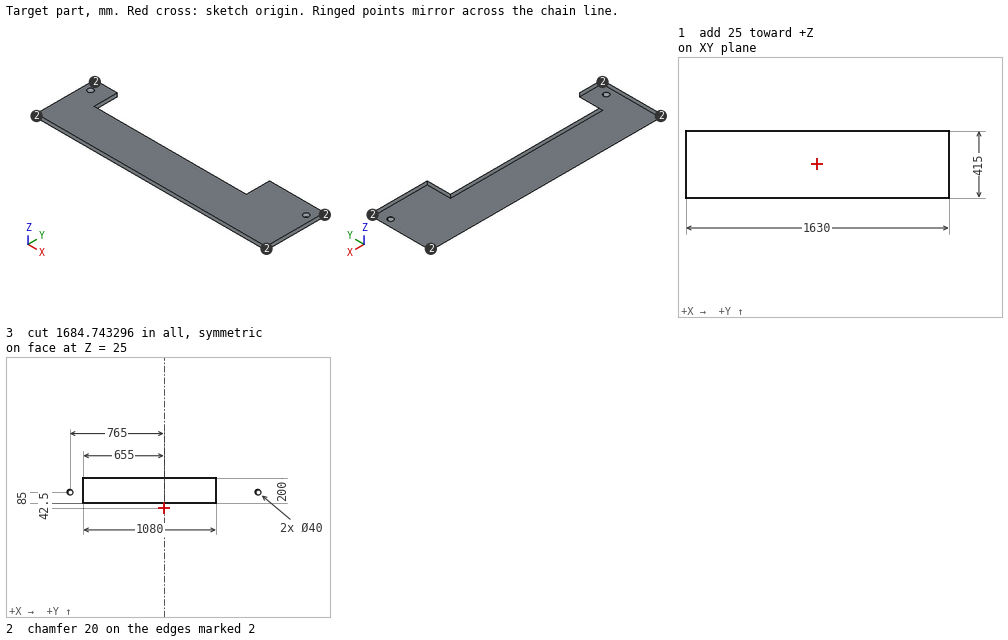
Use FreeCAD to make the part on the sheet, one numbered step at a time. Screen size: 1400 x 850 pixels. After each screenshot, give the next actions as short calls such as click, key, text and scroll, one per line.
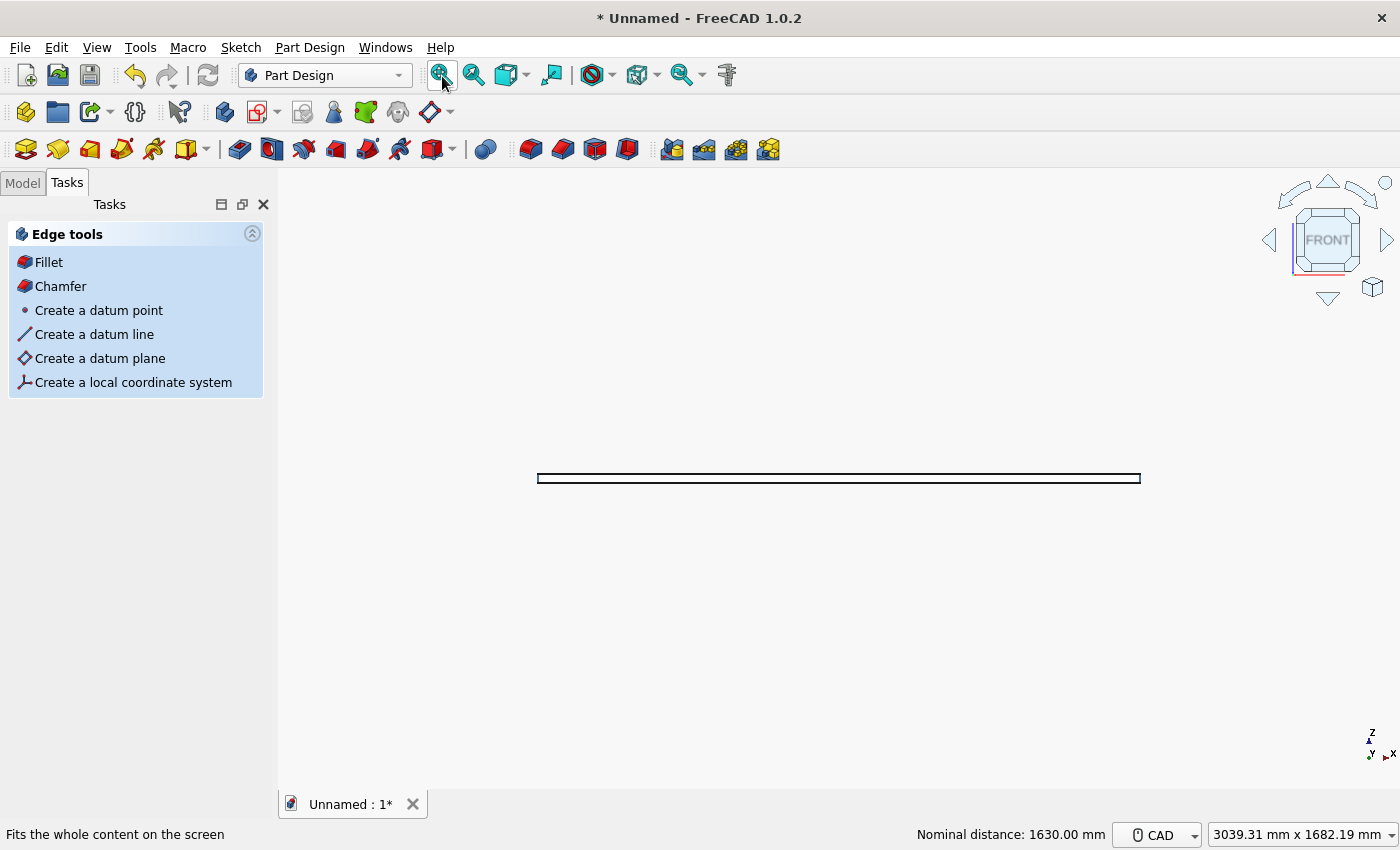
key(3)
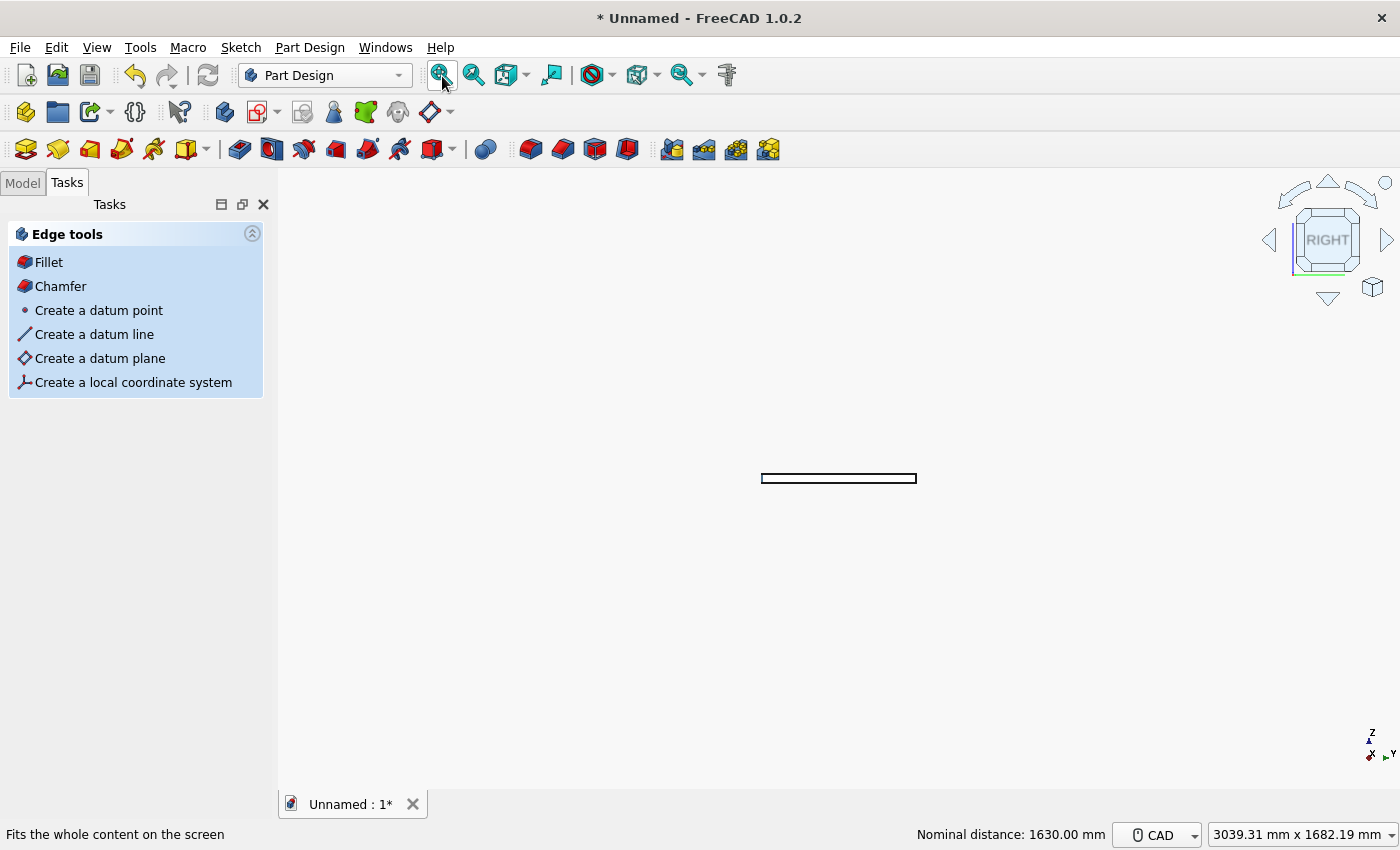
click(442, 76)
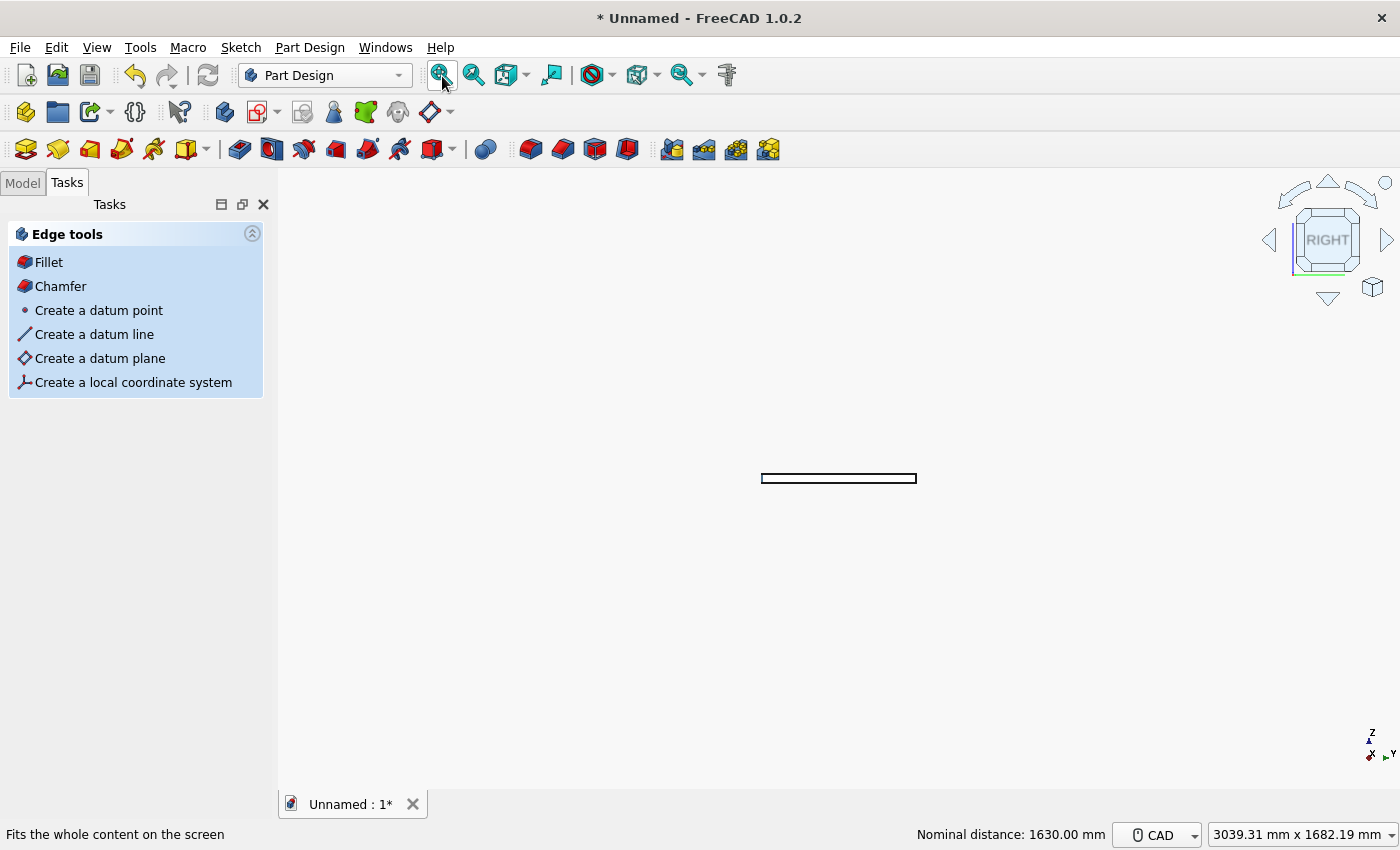
scroll(916, 477, up, 8)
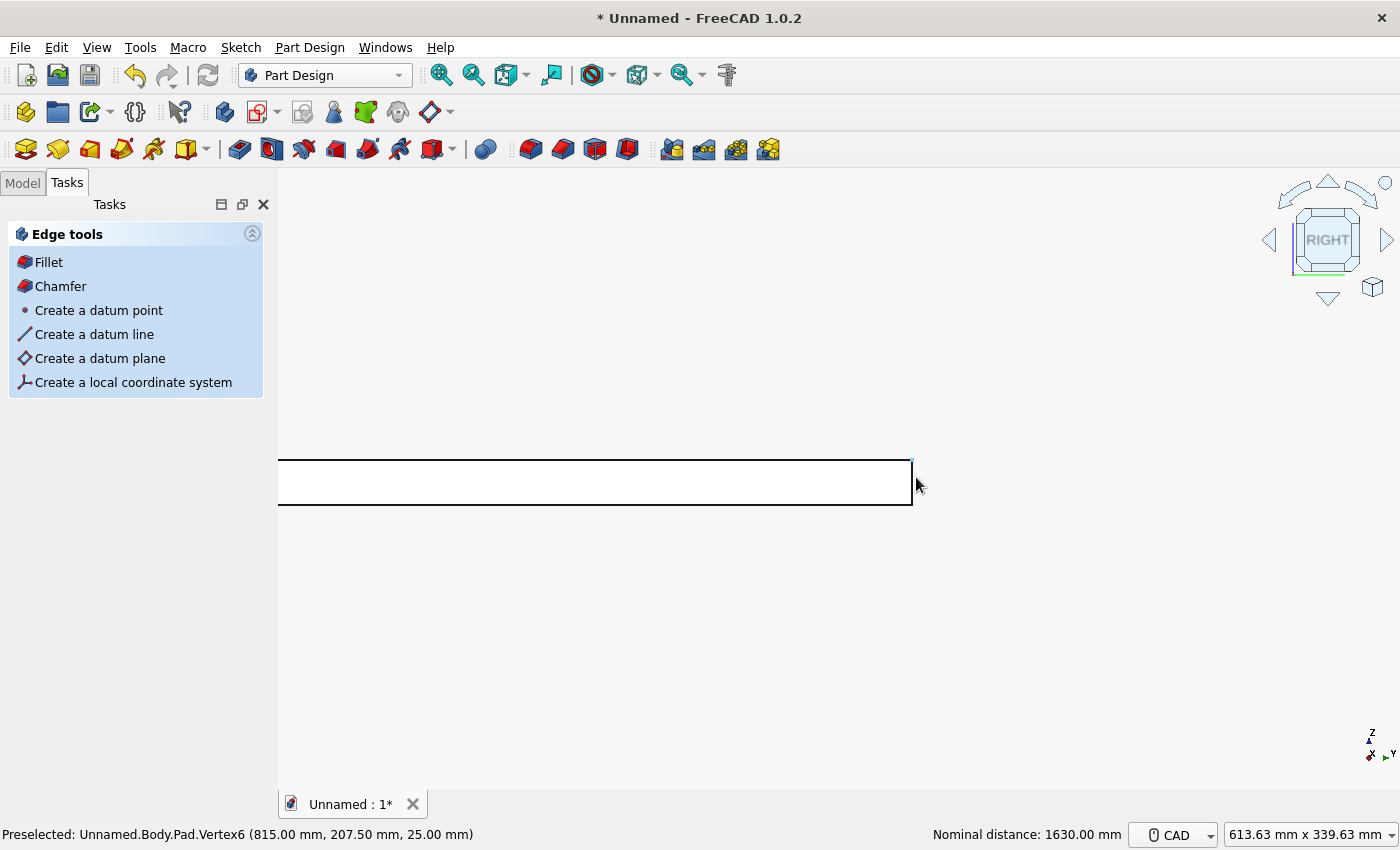
click(912, 481, ctrl)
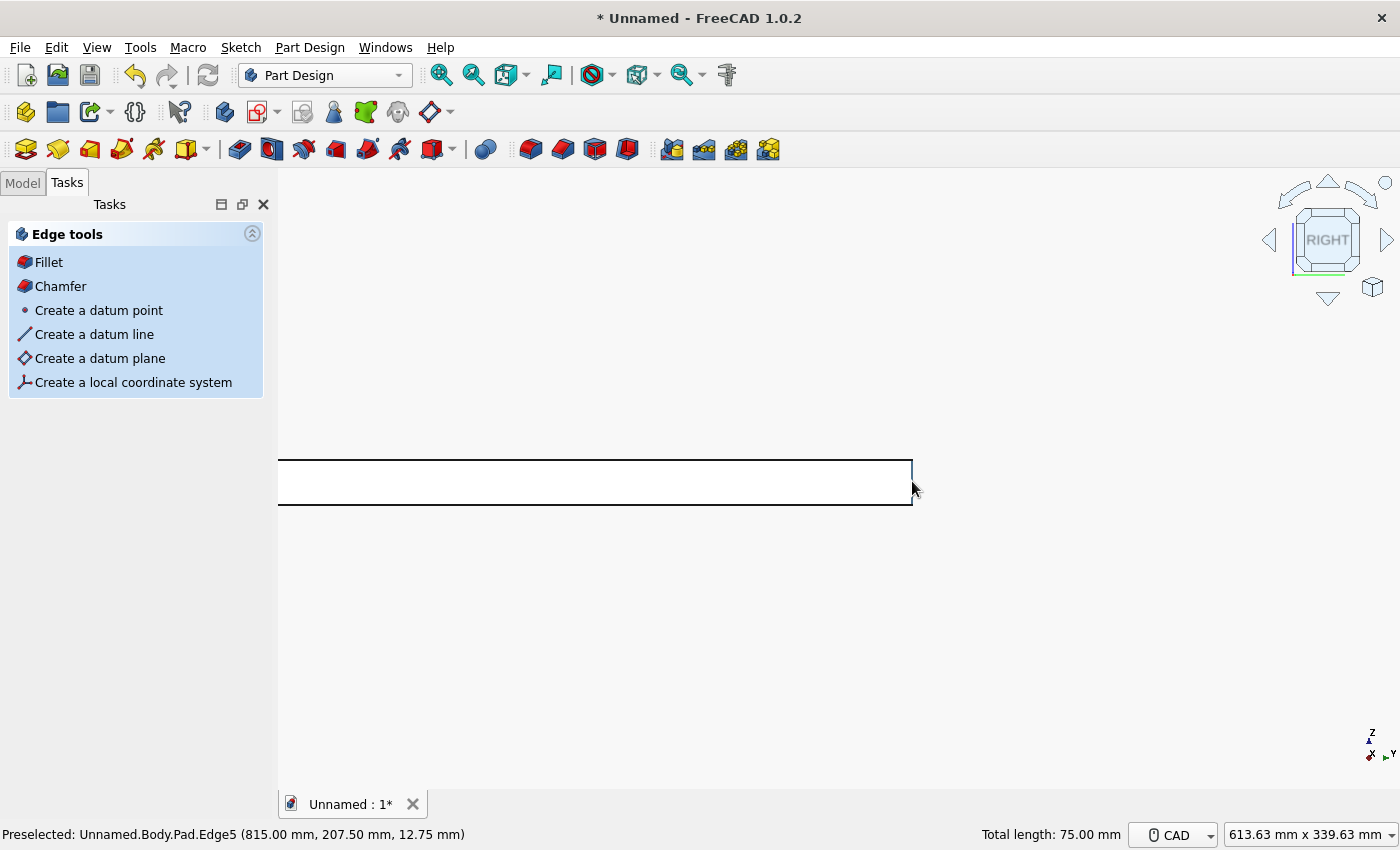
click(442, 76)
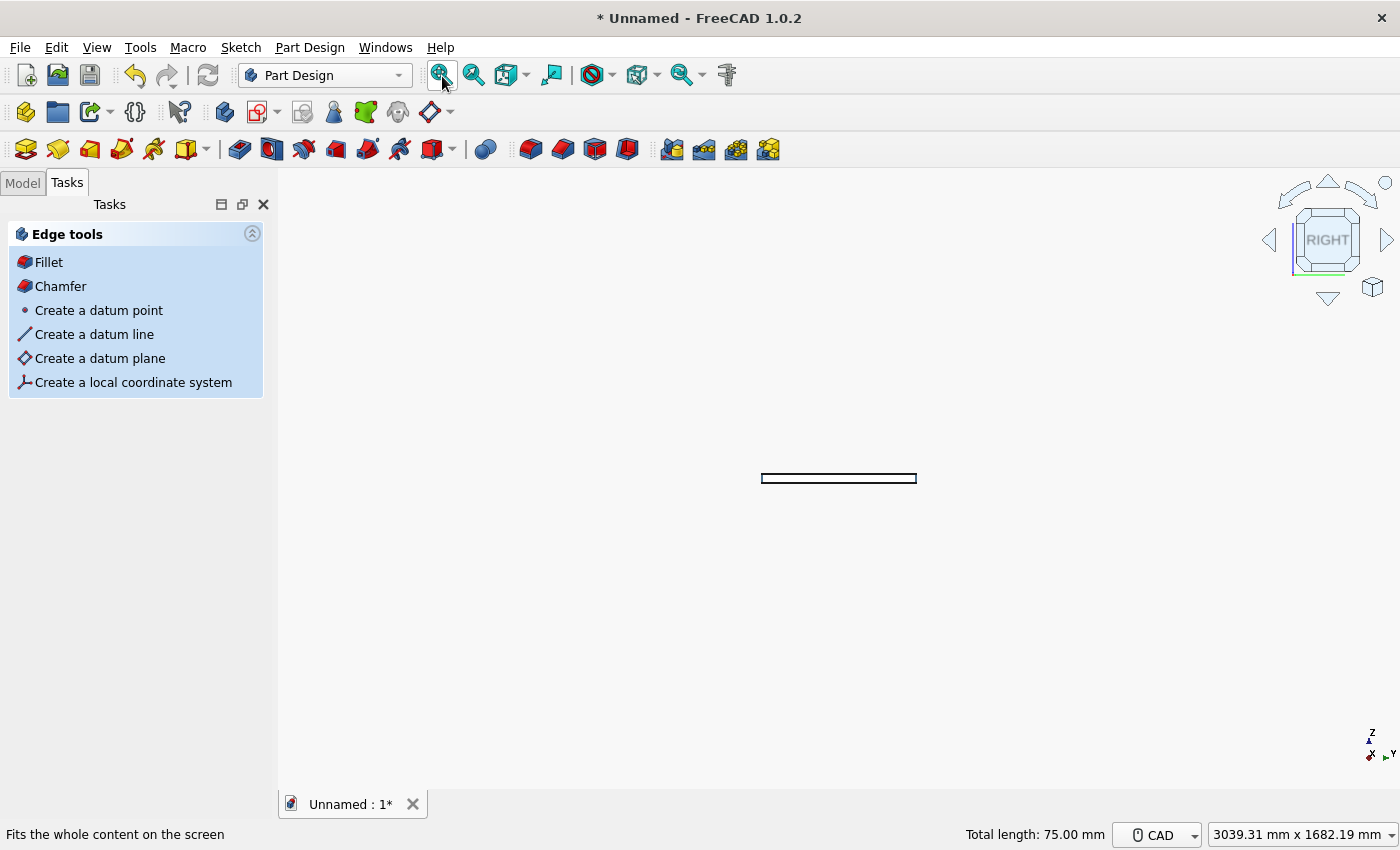
key(5)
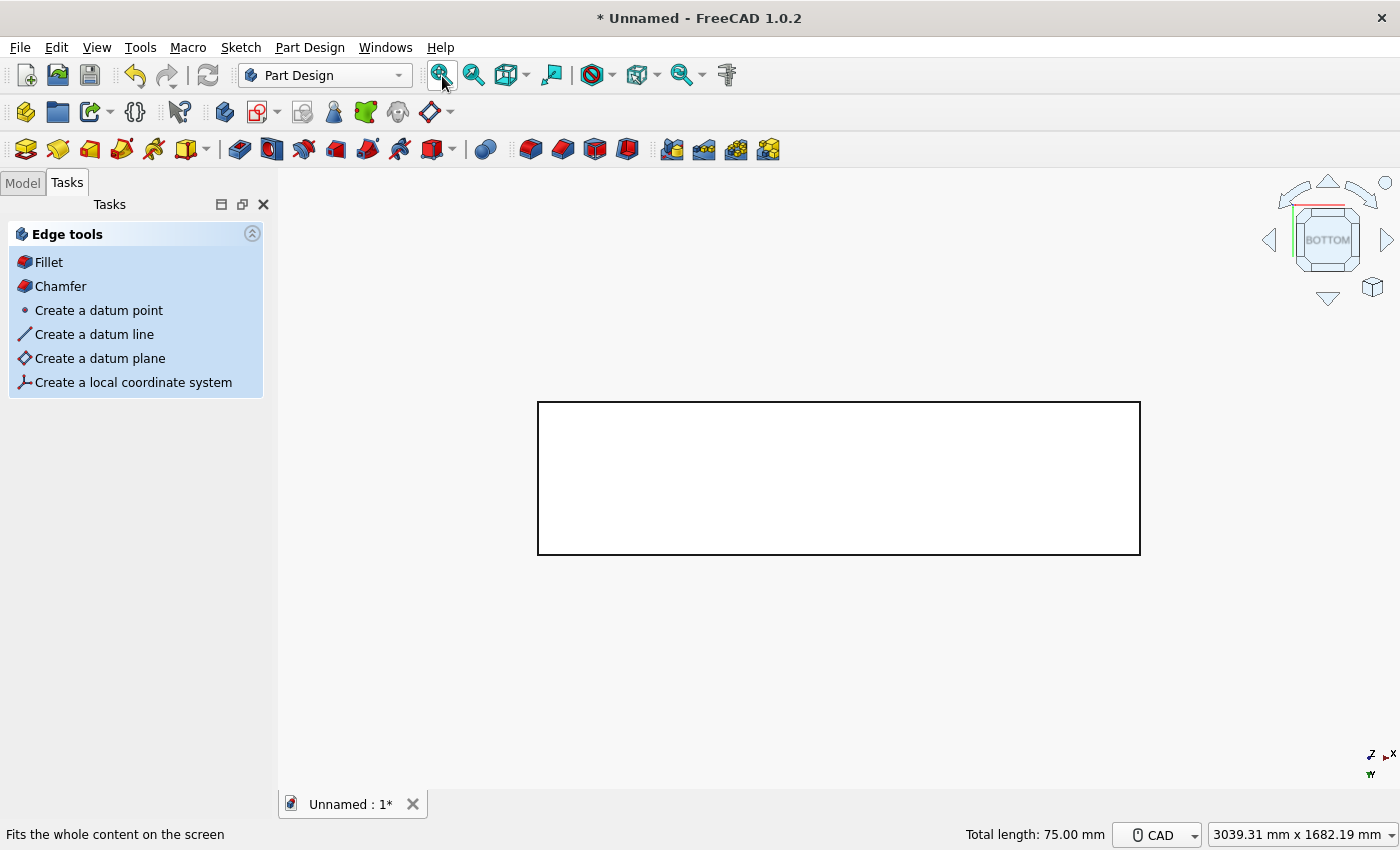
scroll(538, 554, up, 8)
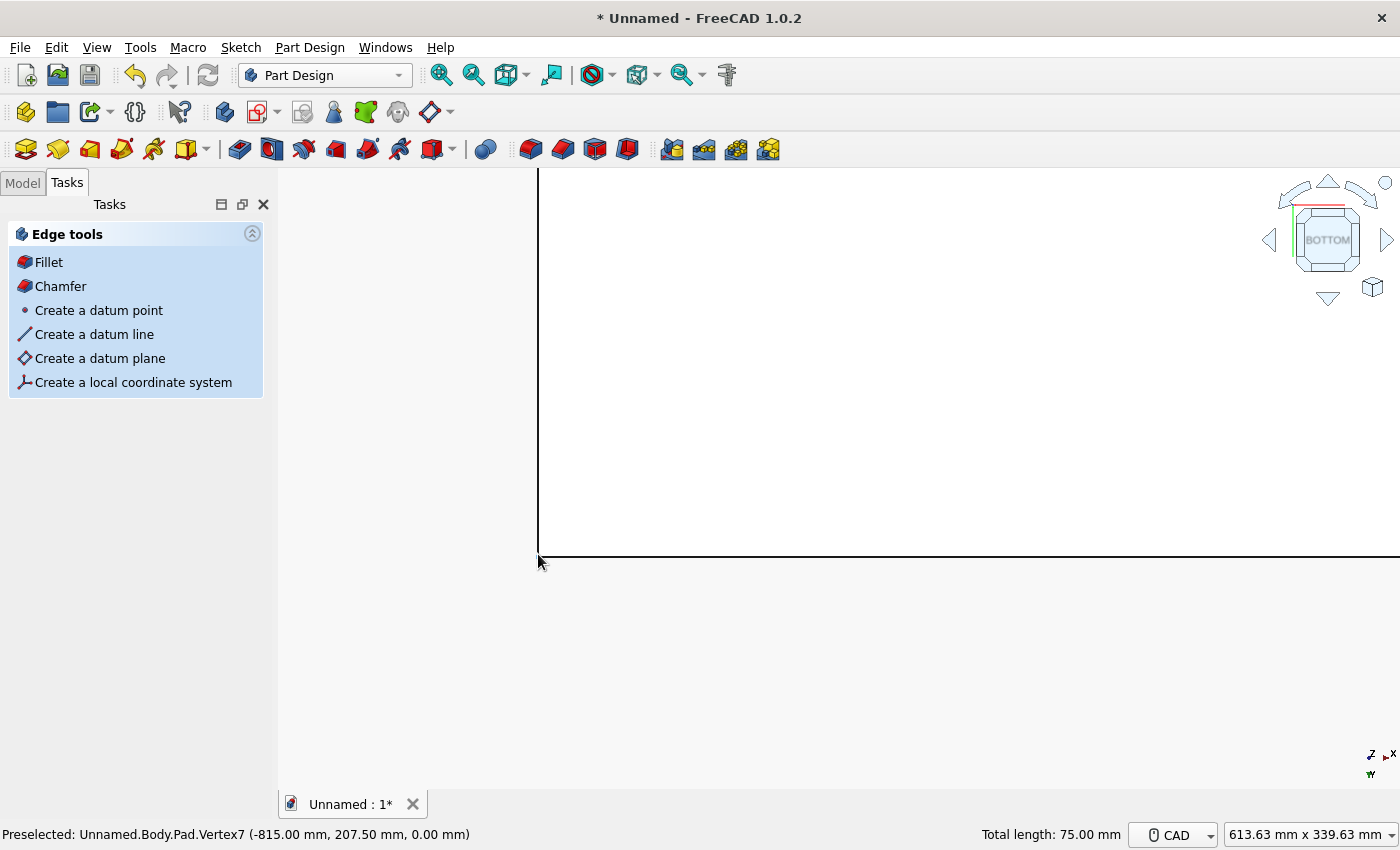
click(442, 76)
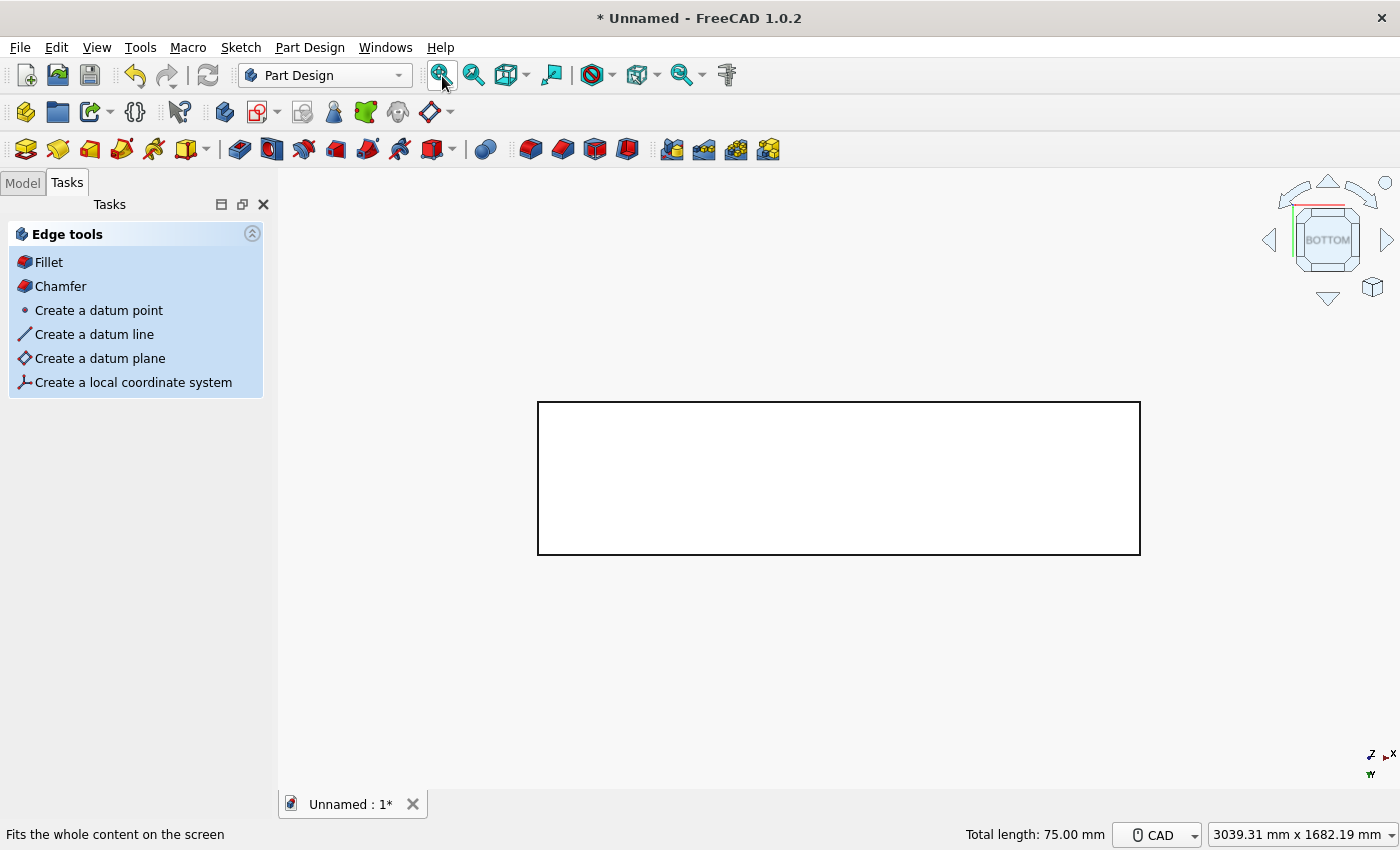
key(4)